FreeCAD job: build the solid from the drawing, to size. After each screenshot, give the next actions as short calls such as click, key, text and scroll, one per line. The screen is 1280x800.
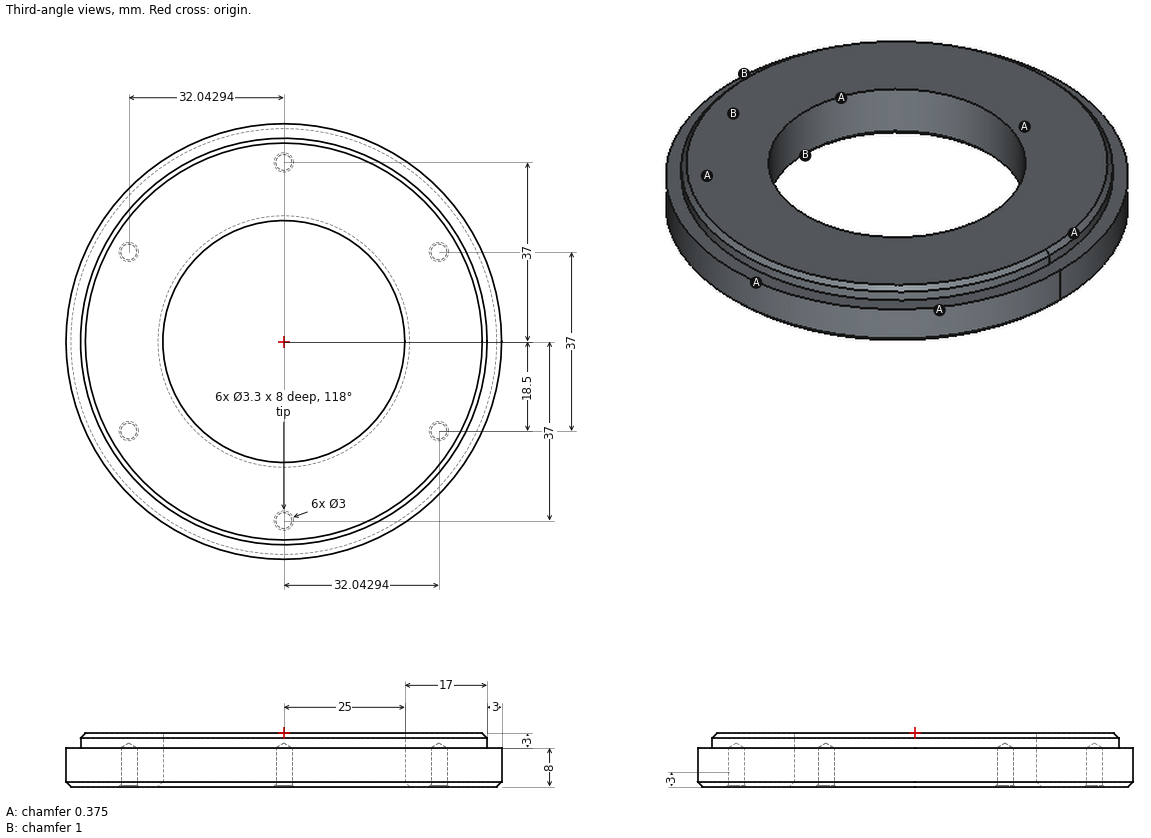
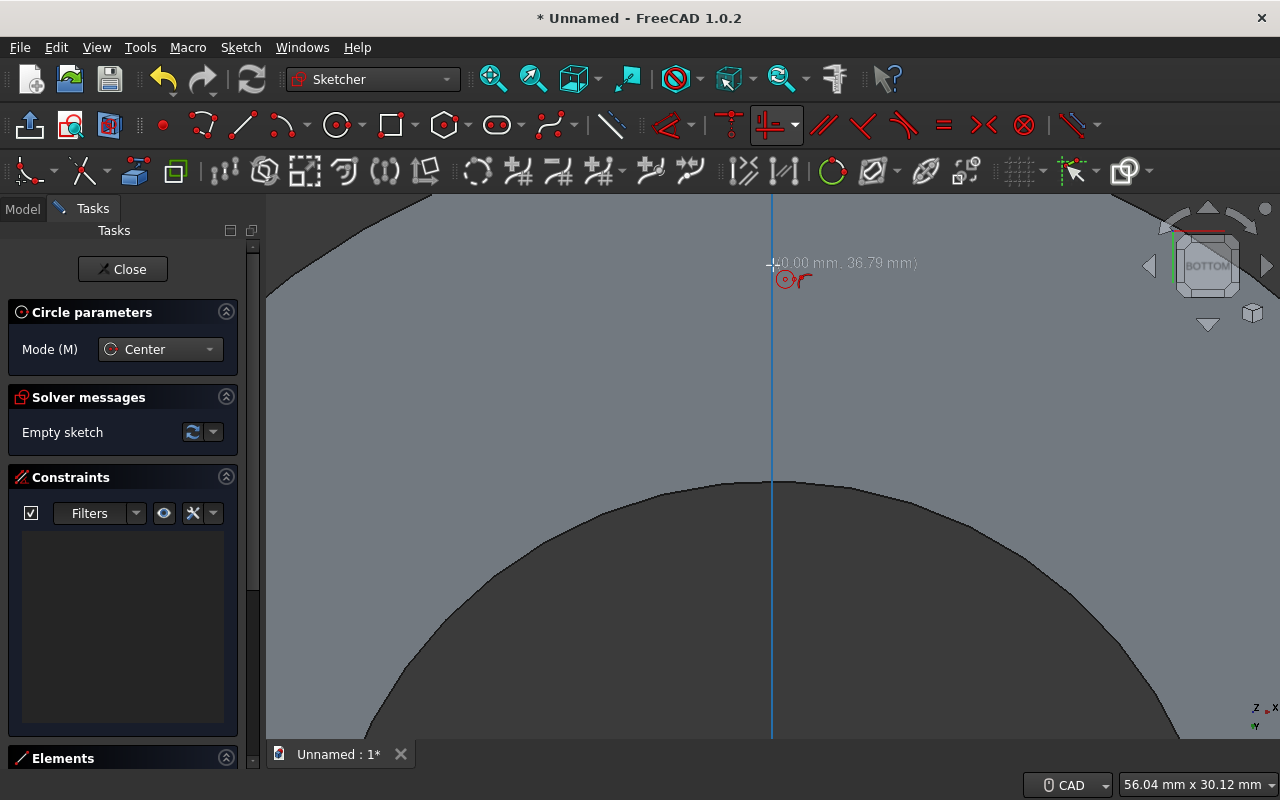
click(772, 264)
move(791, 245)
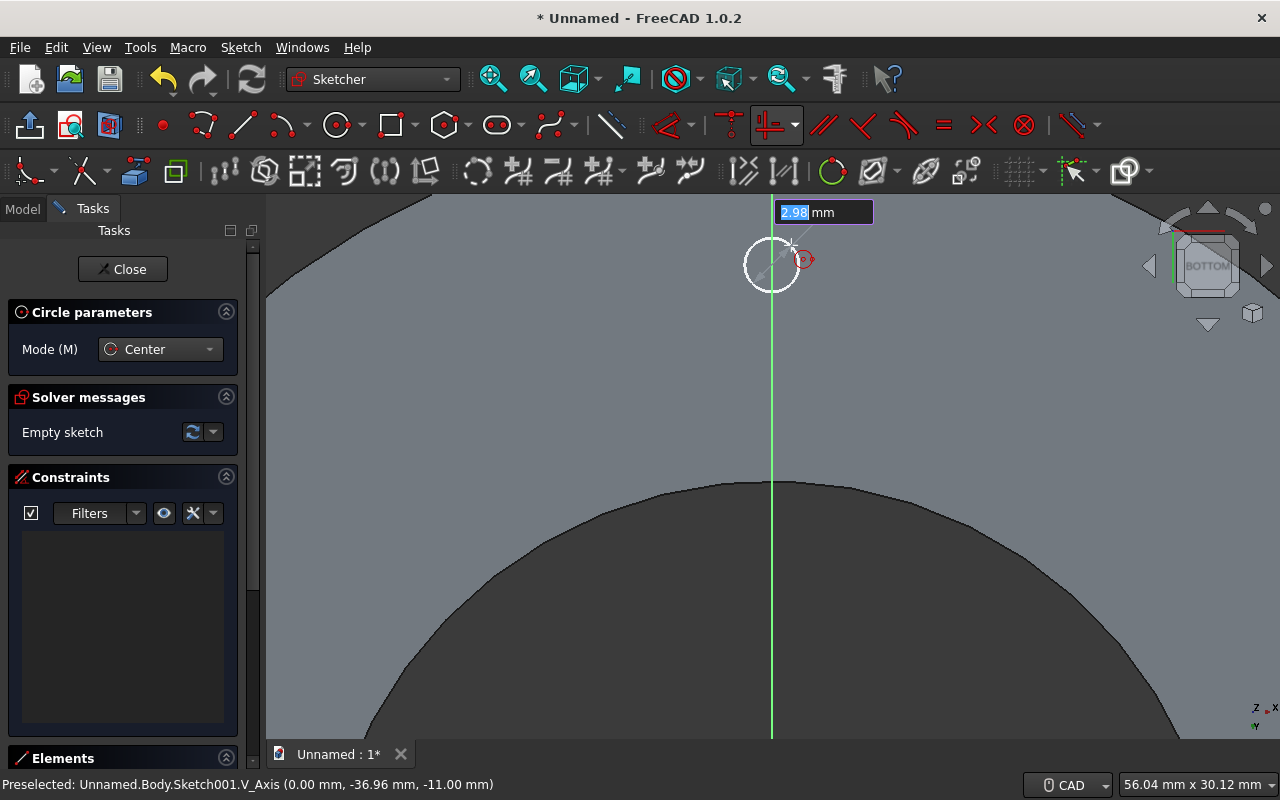
text(3)
key(Return)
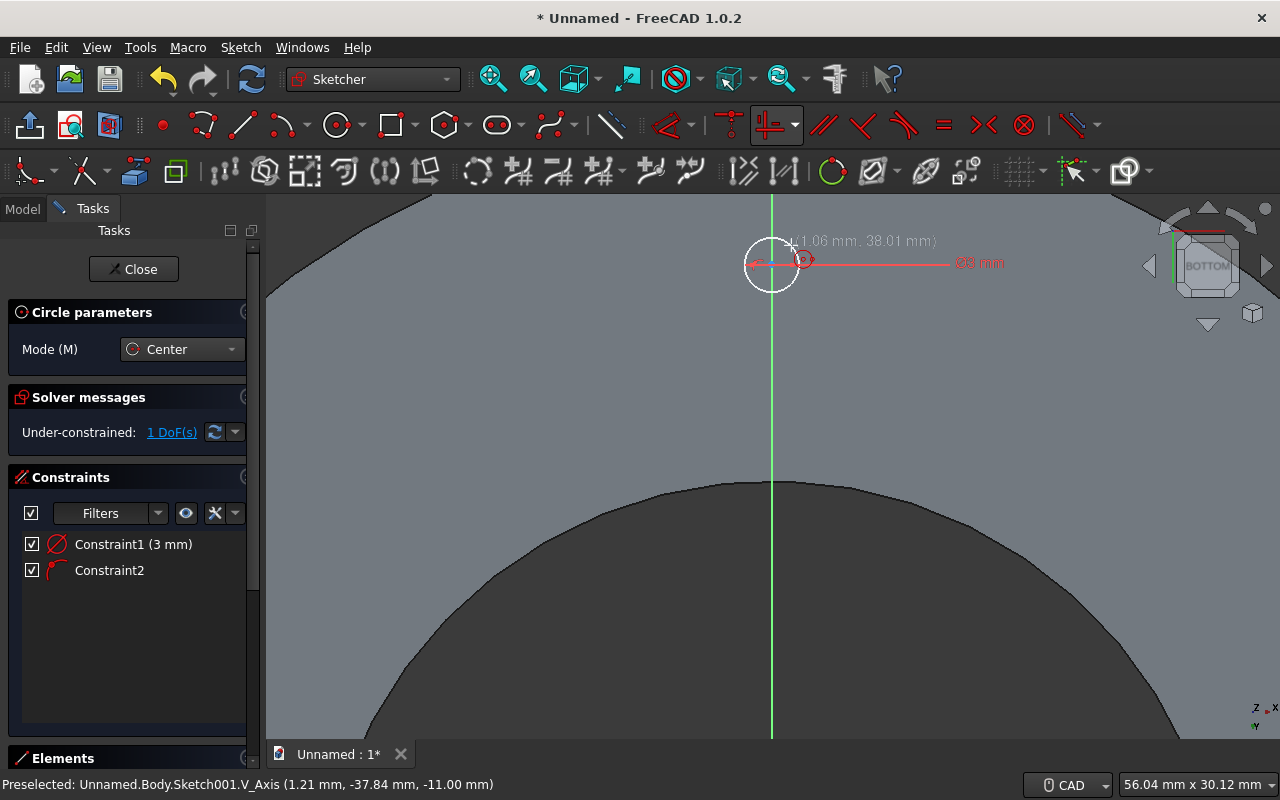
scroll(682, 314, down, 7)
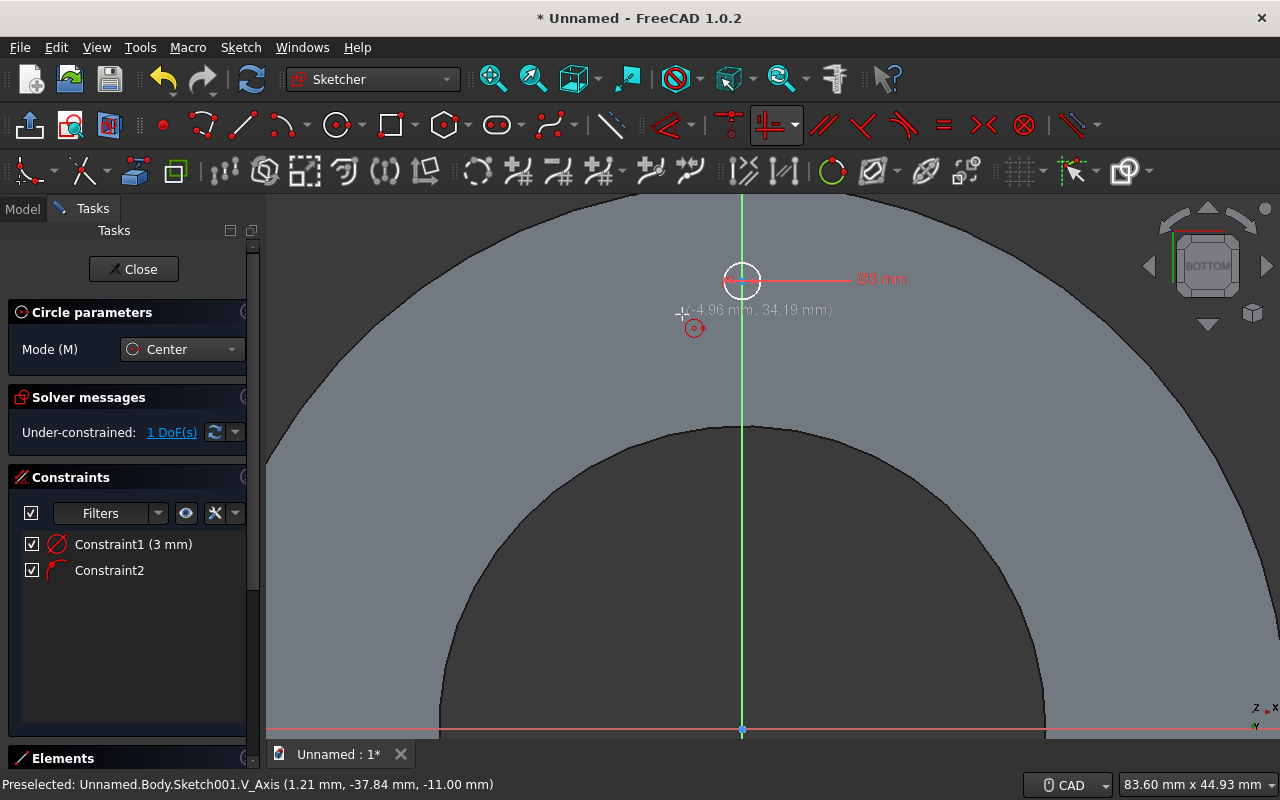
scroll(847, 384, up, 7)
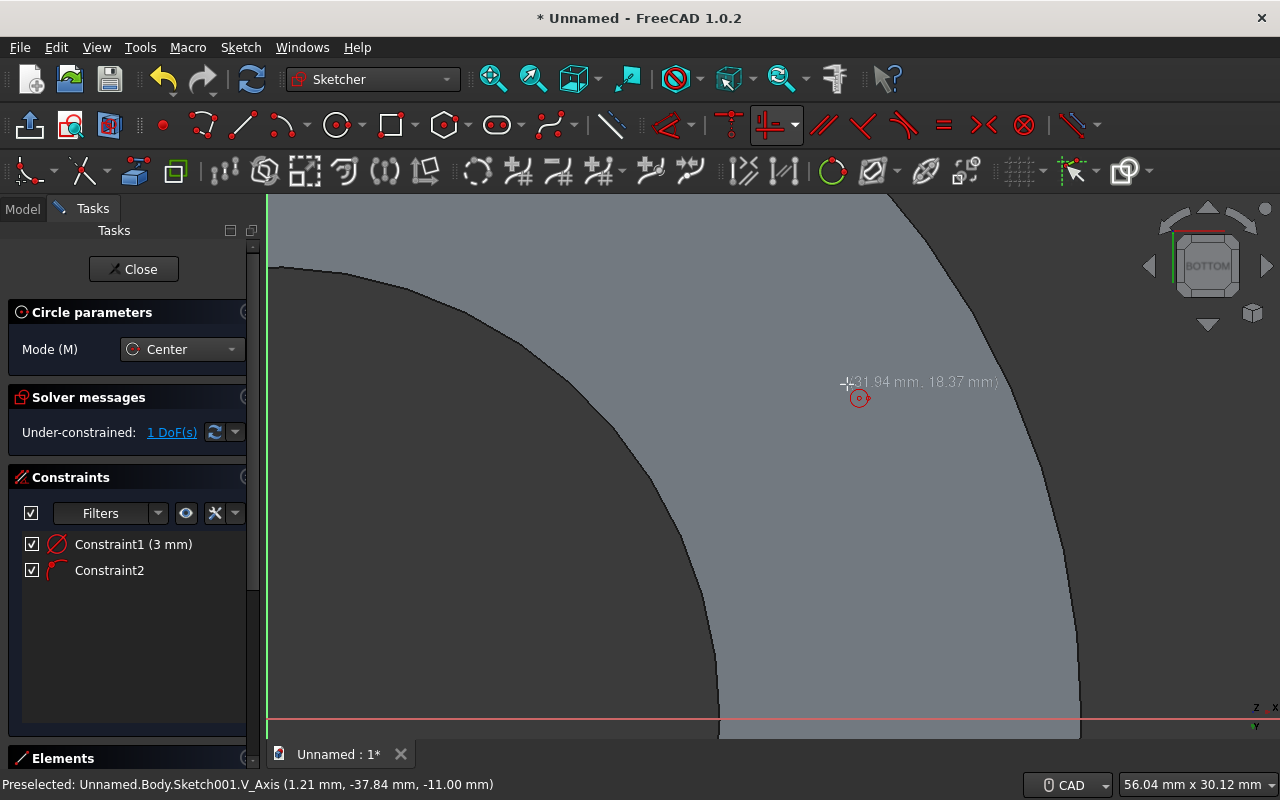
click(847, 385)
move(866, 366)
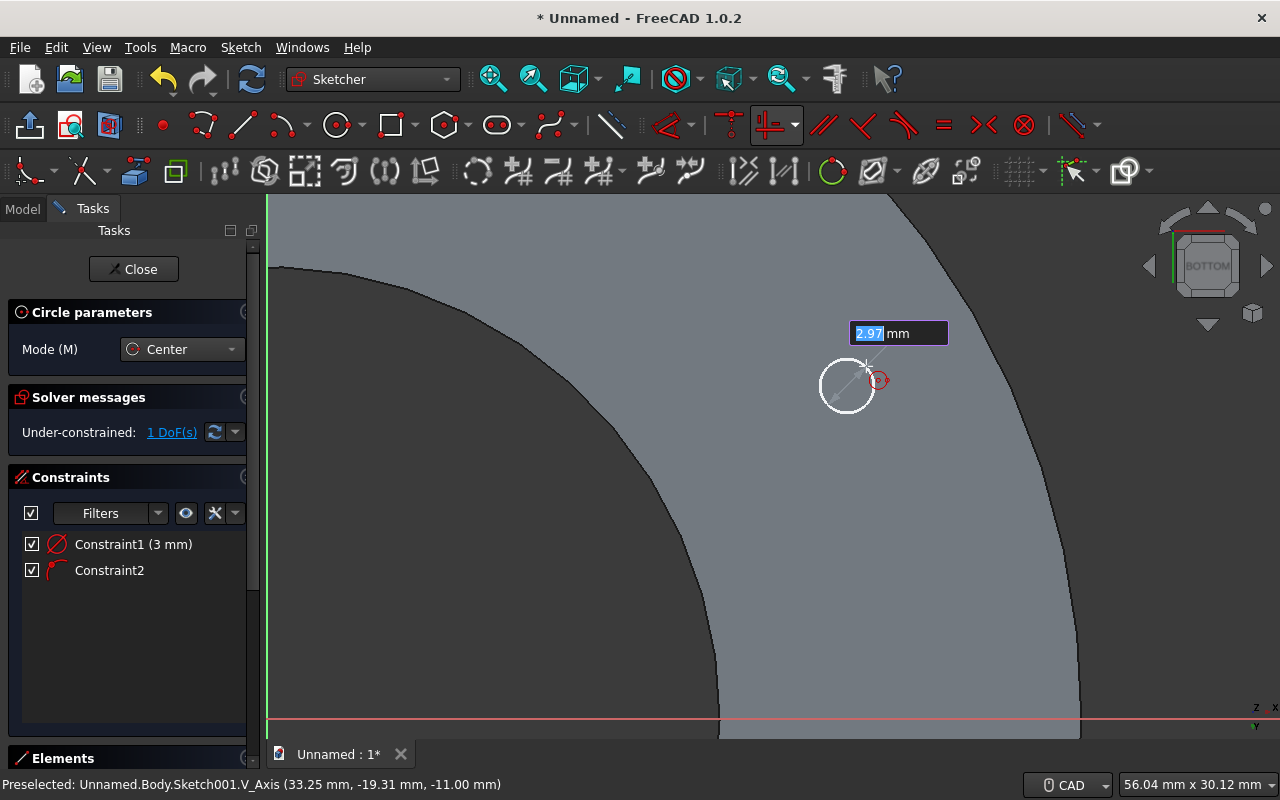
text(3)
key(Return)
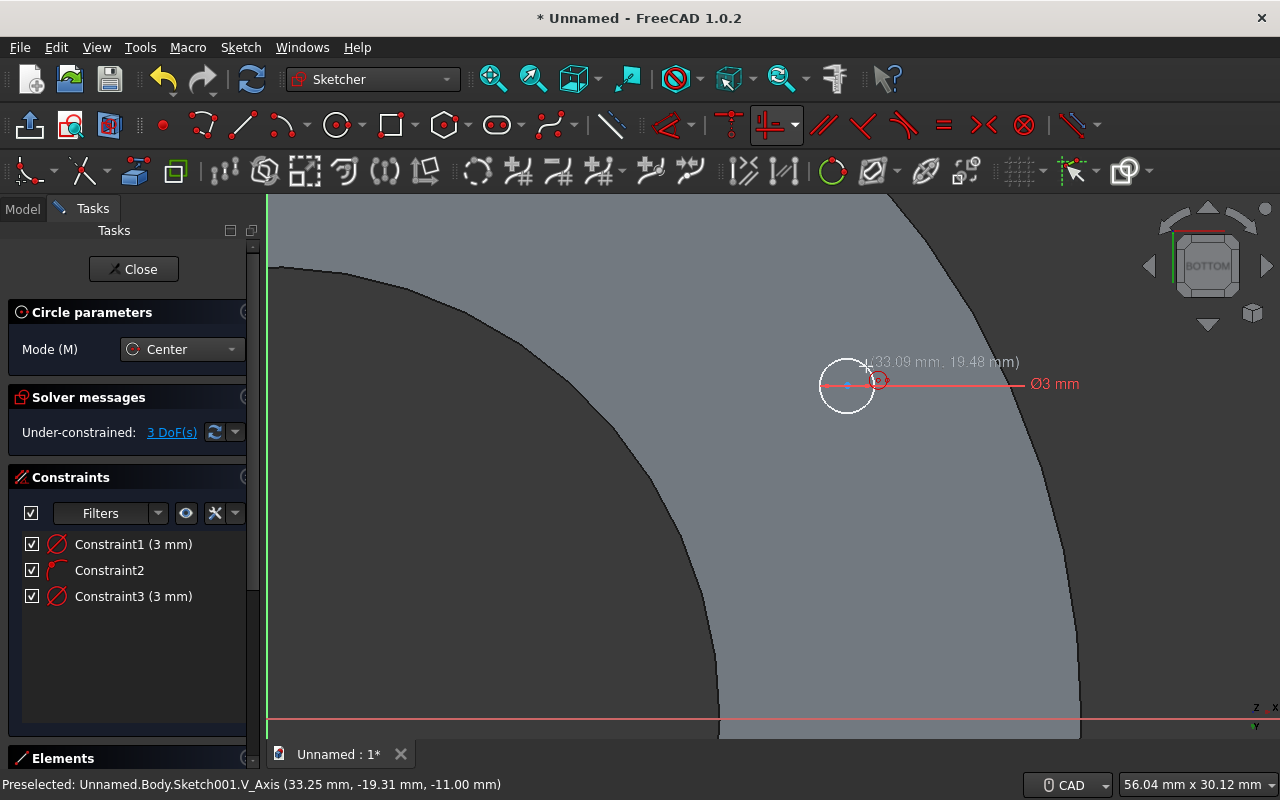
scroll(848, 384, down, 7)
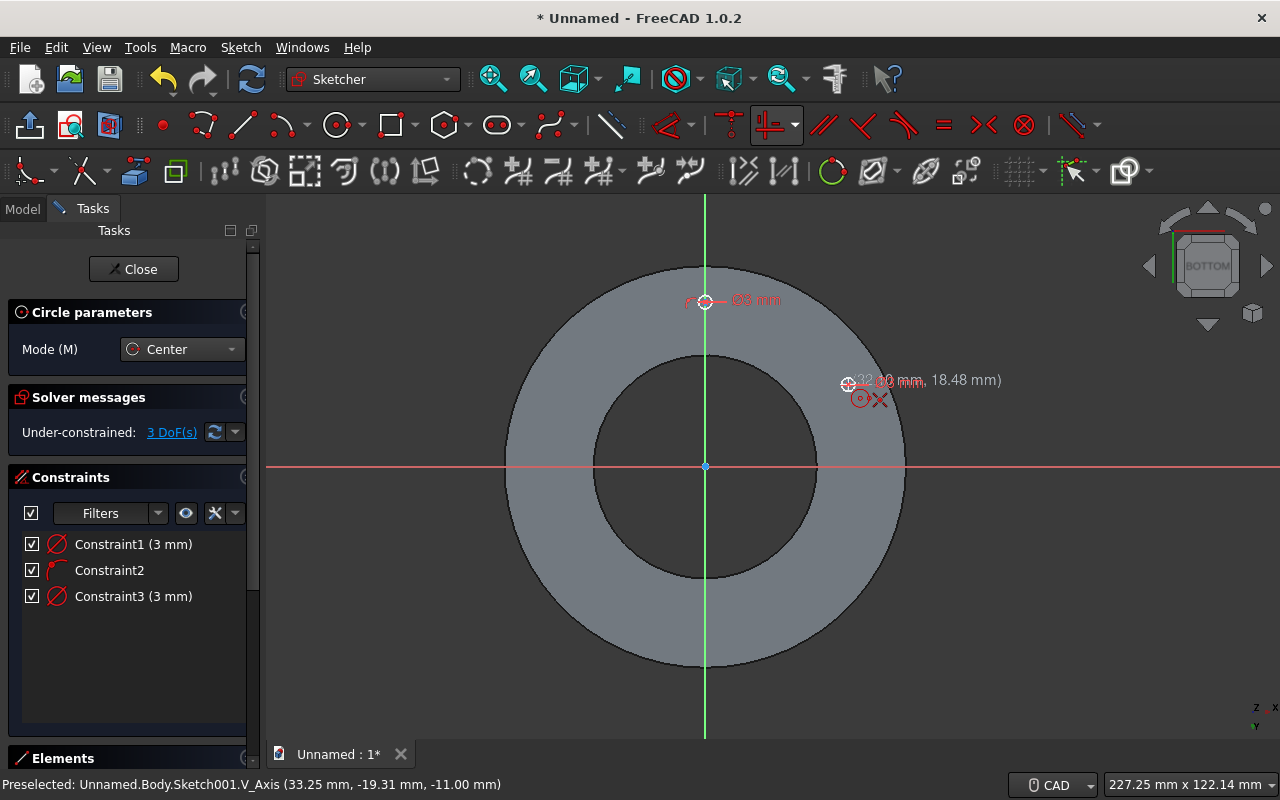
scroll(848, 550, up, 7)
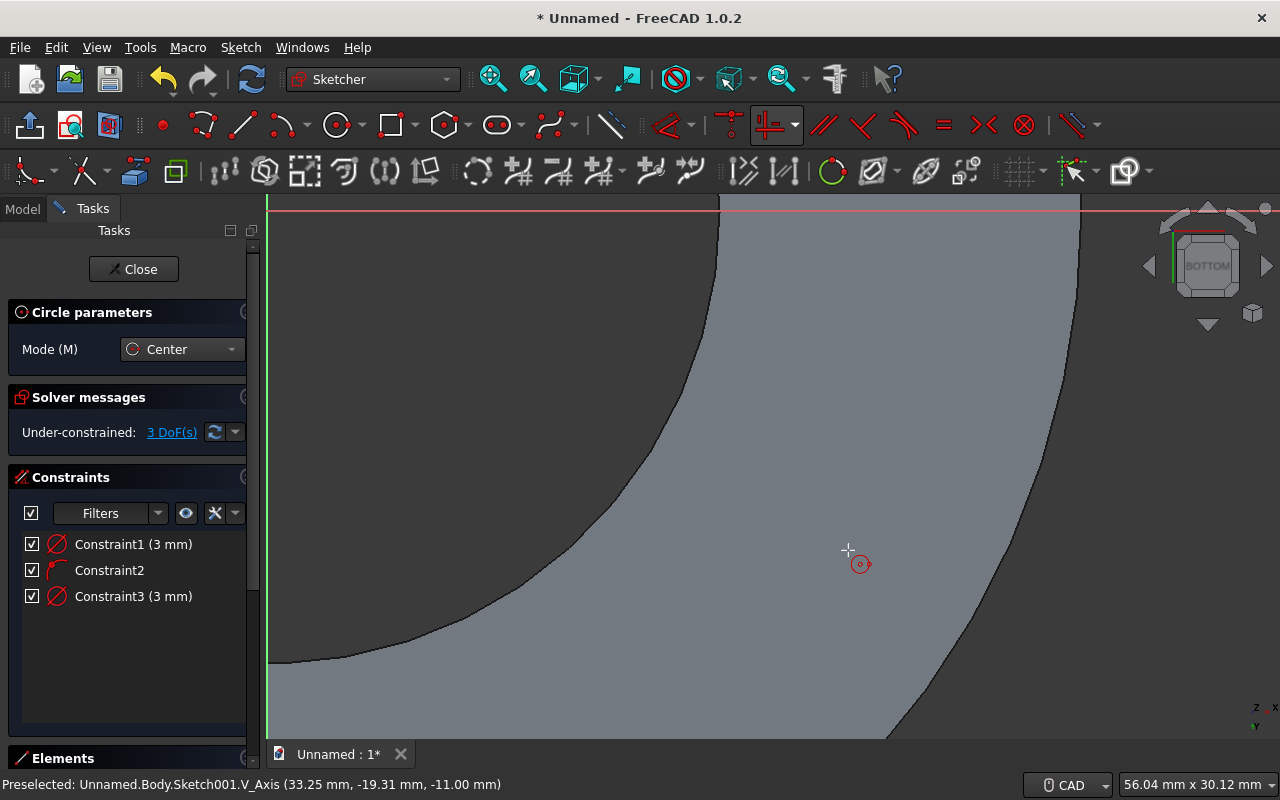
click(847, 546)
move(866, 527)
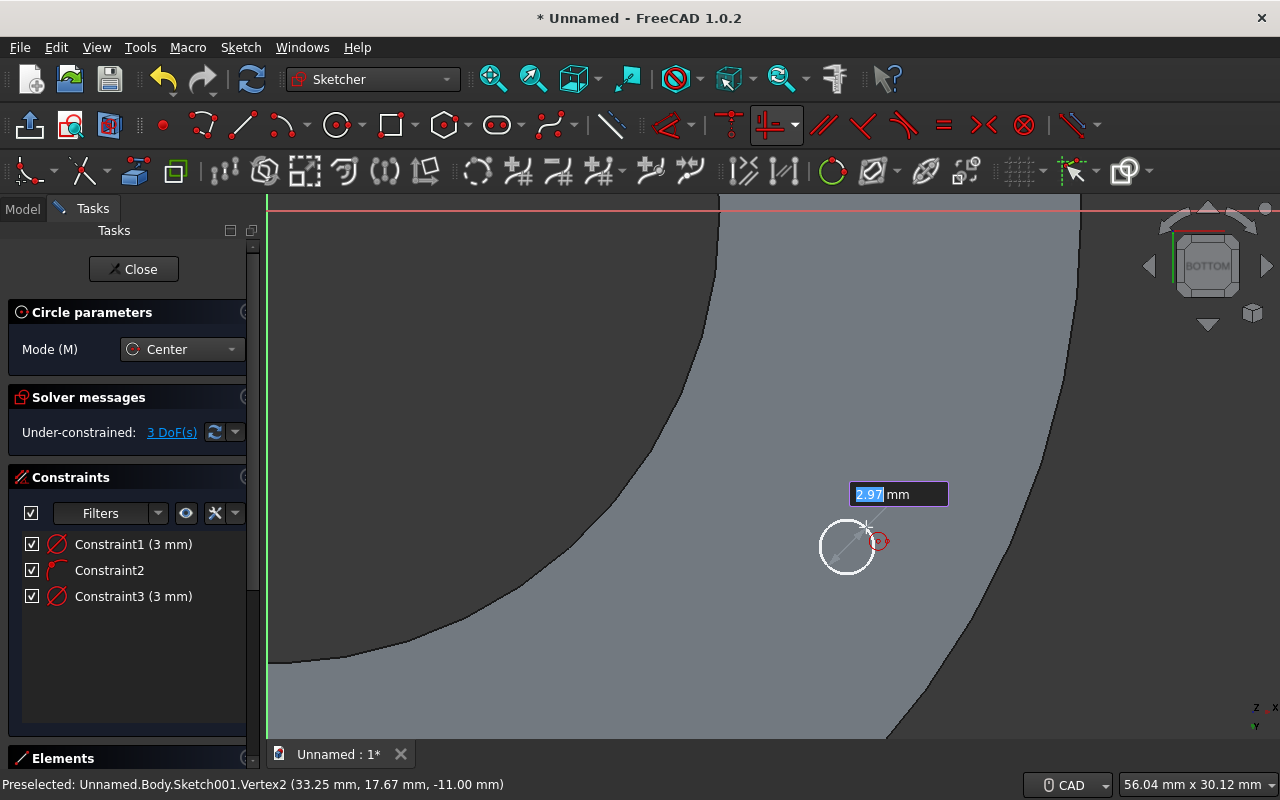
text(3)
key(Return)